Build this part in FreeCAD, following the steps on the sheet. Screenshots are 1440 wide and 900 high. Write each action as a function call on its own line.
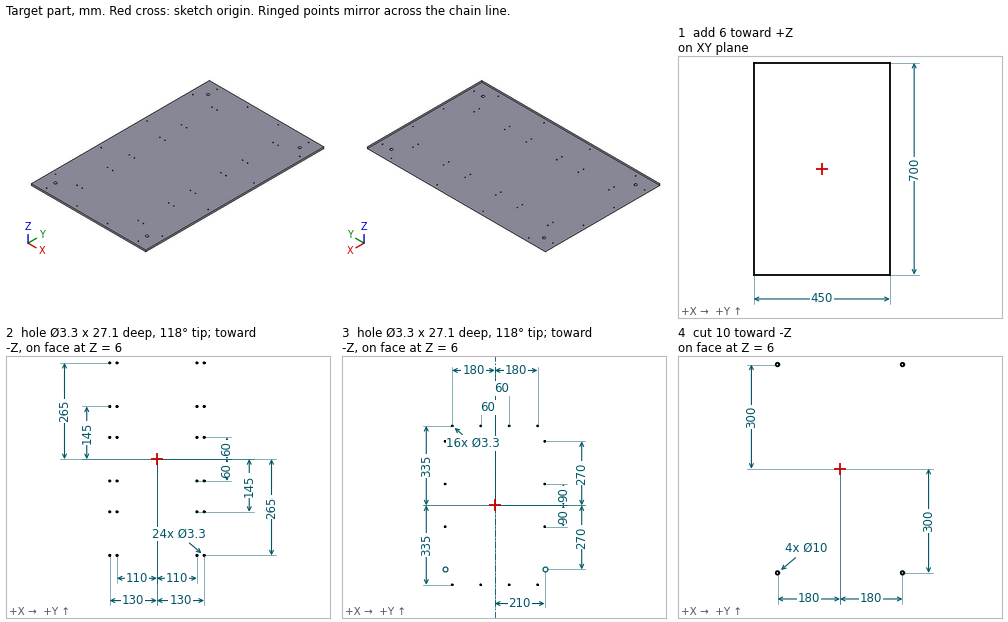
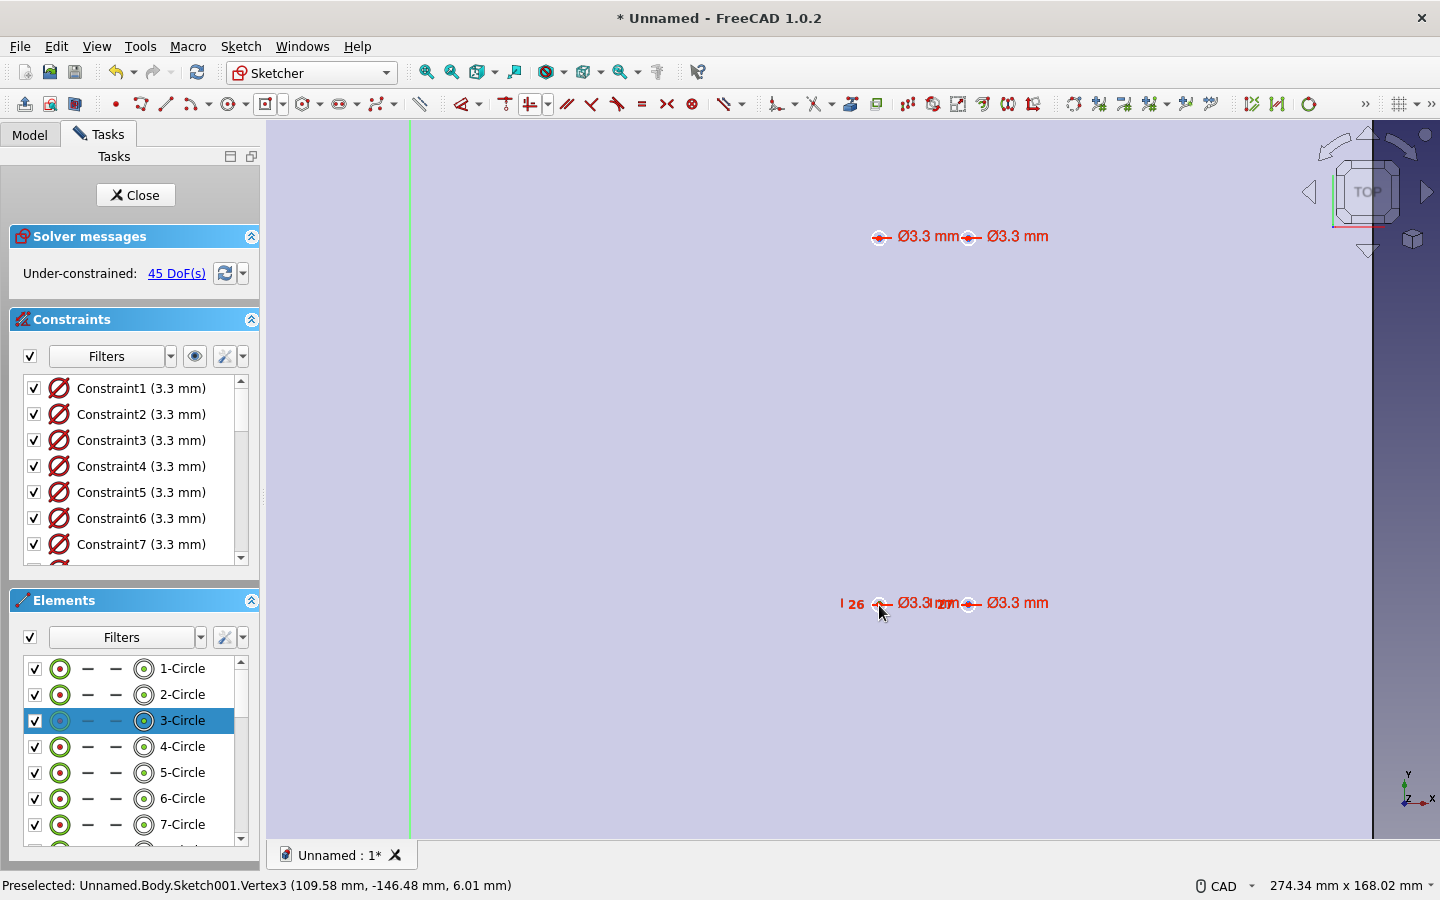
scroll(879, 606, down, 8)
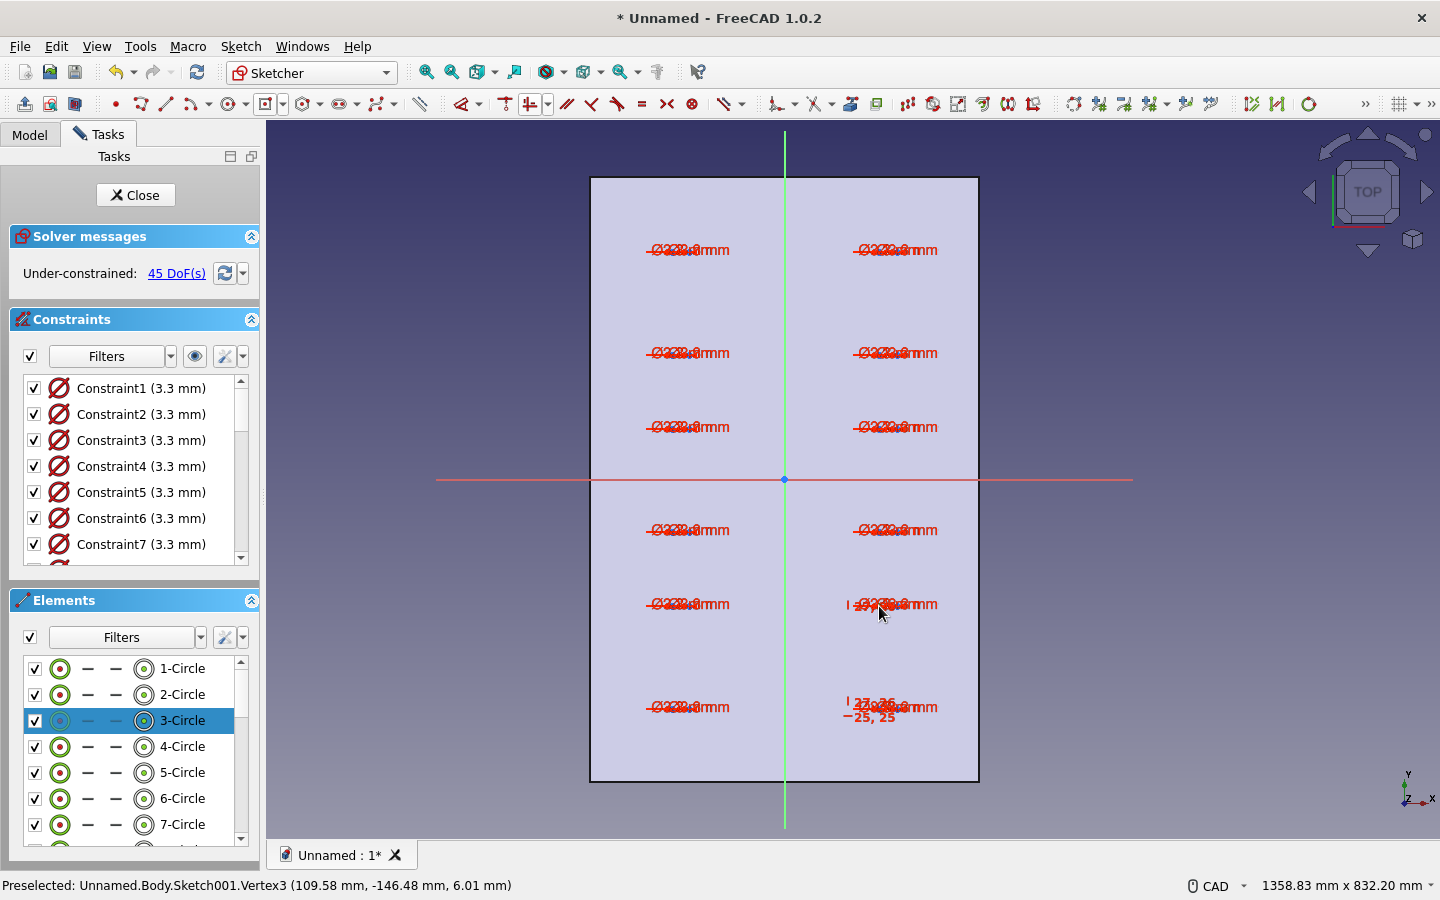
click(897, 606)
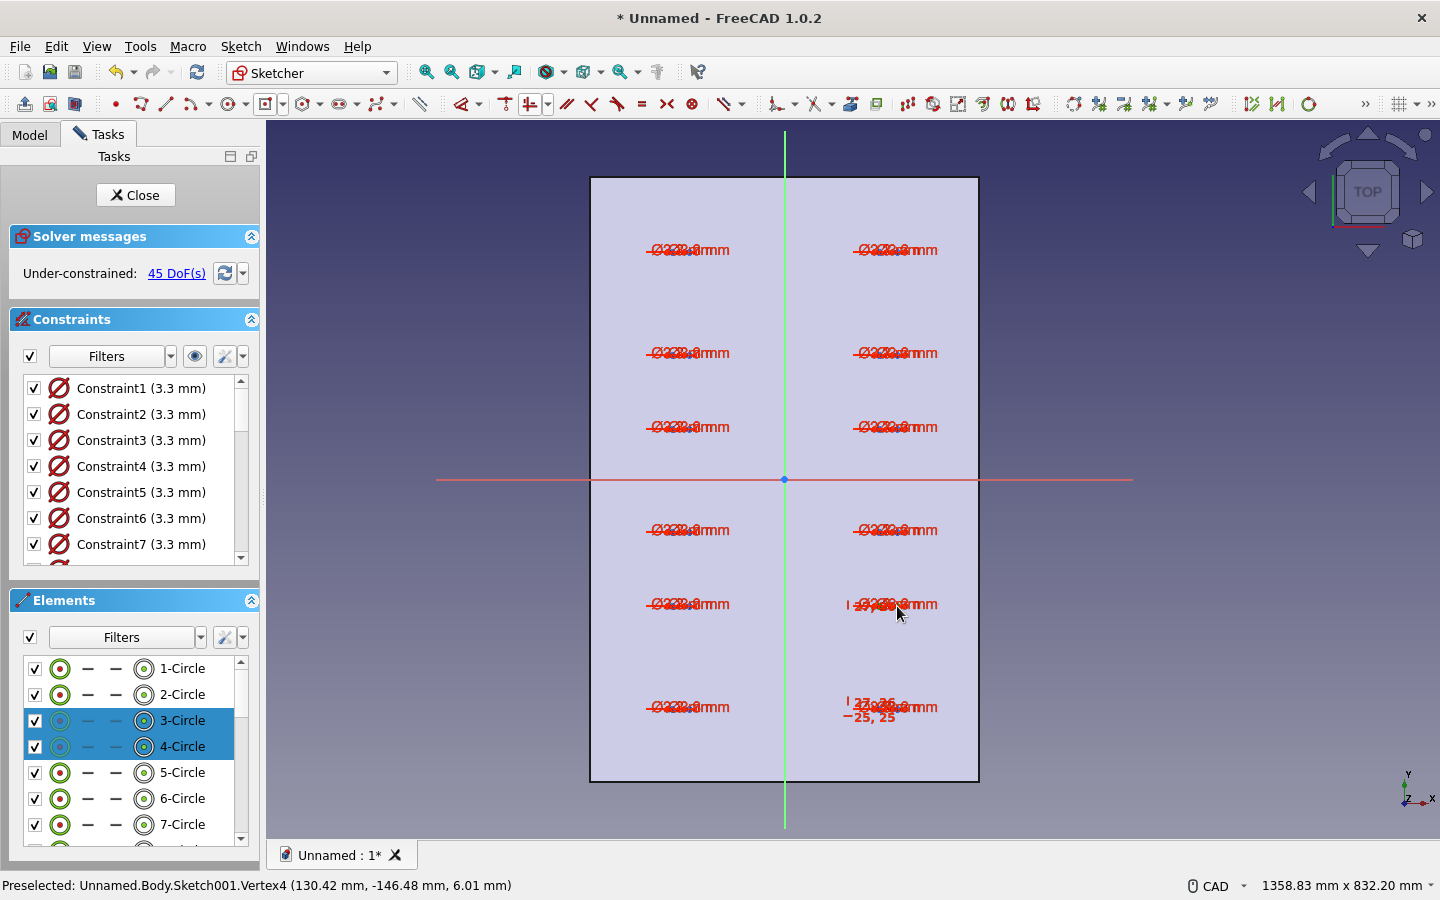
click(548, 104)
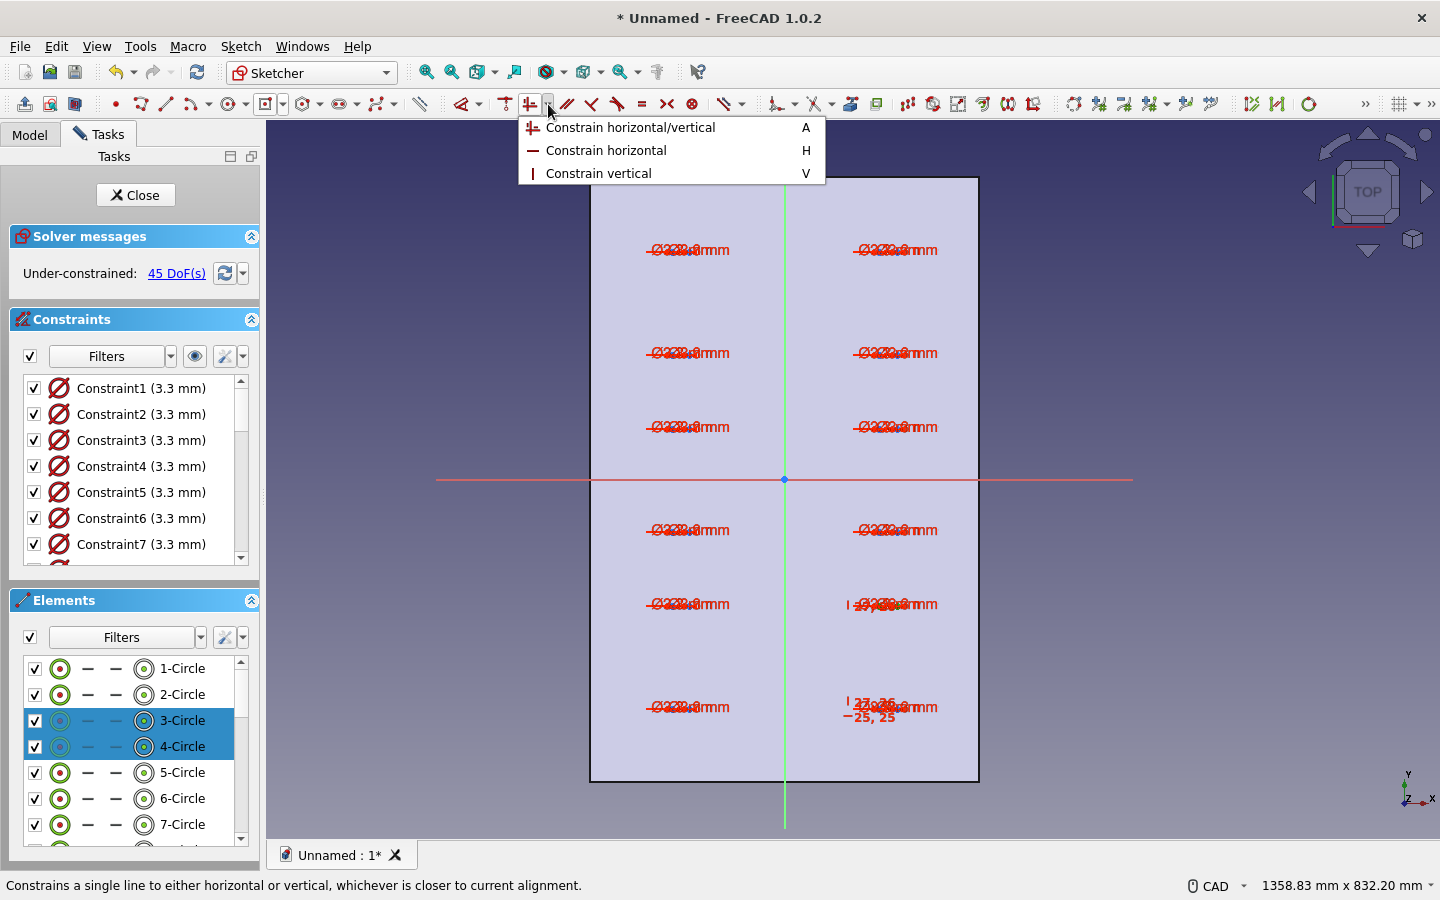
click(672, 150)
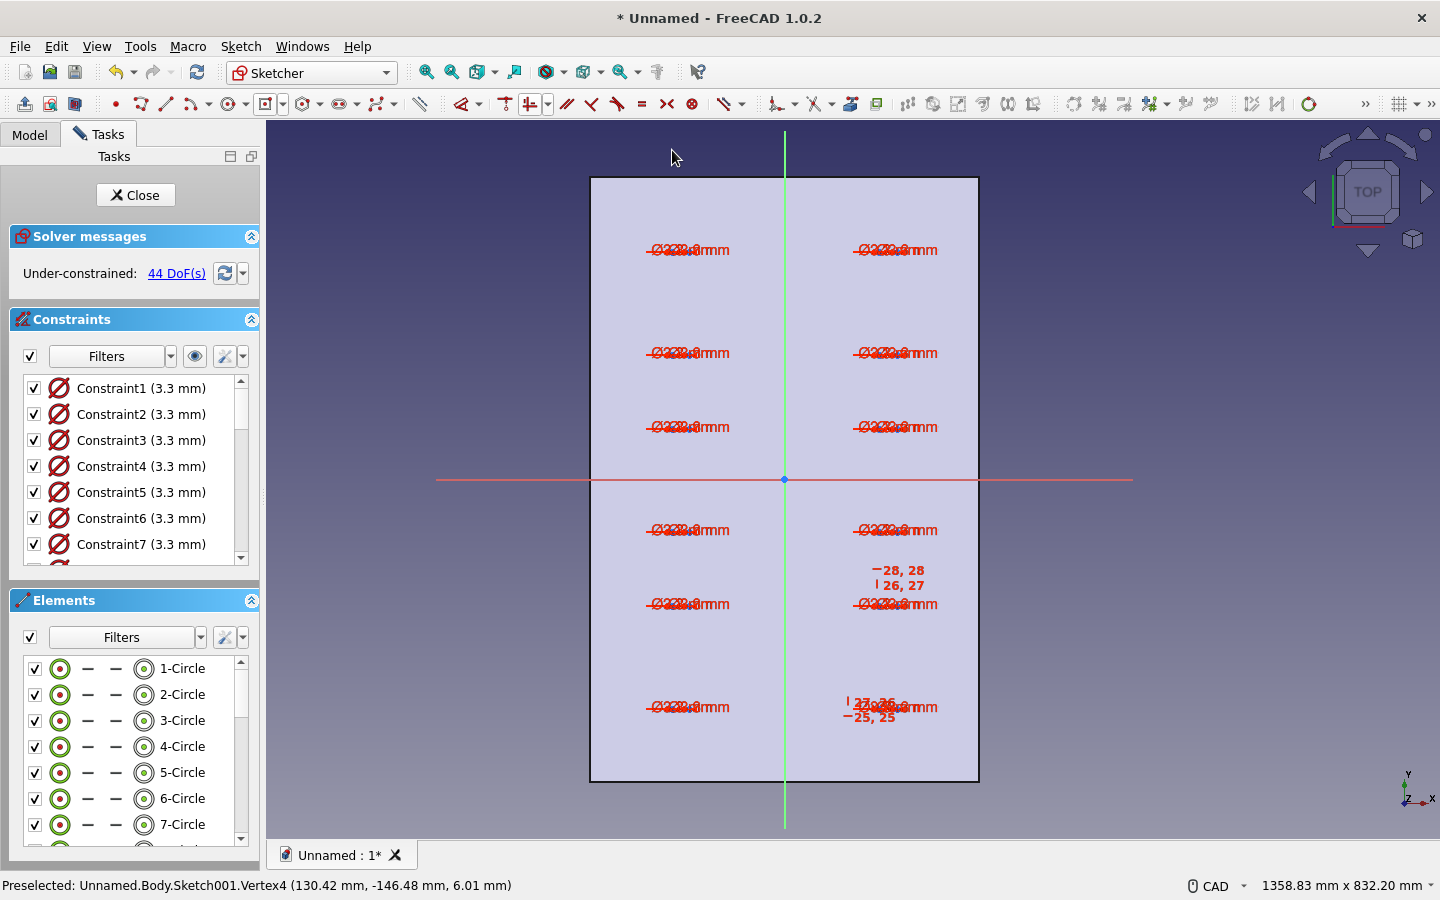
click(879, 606)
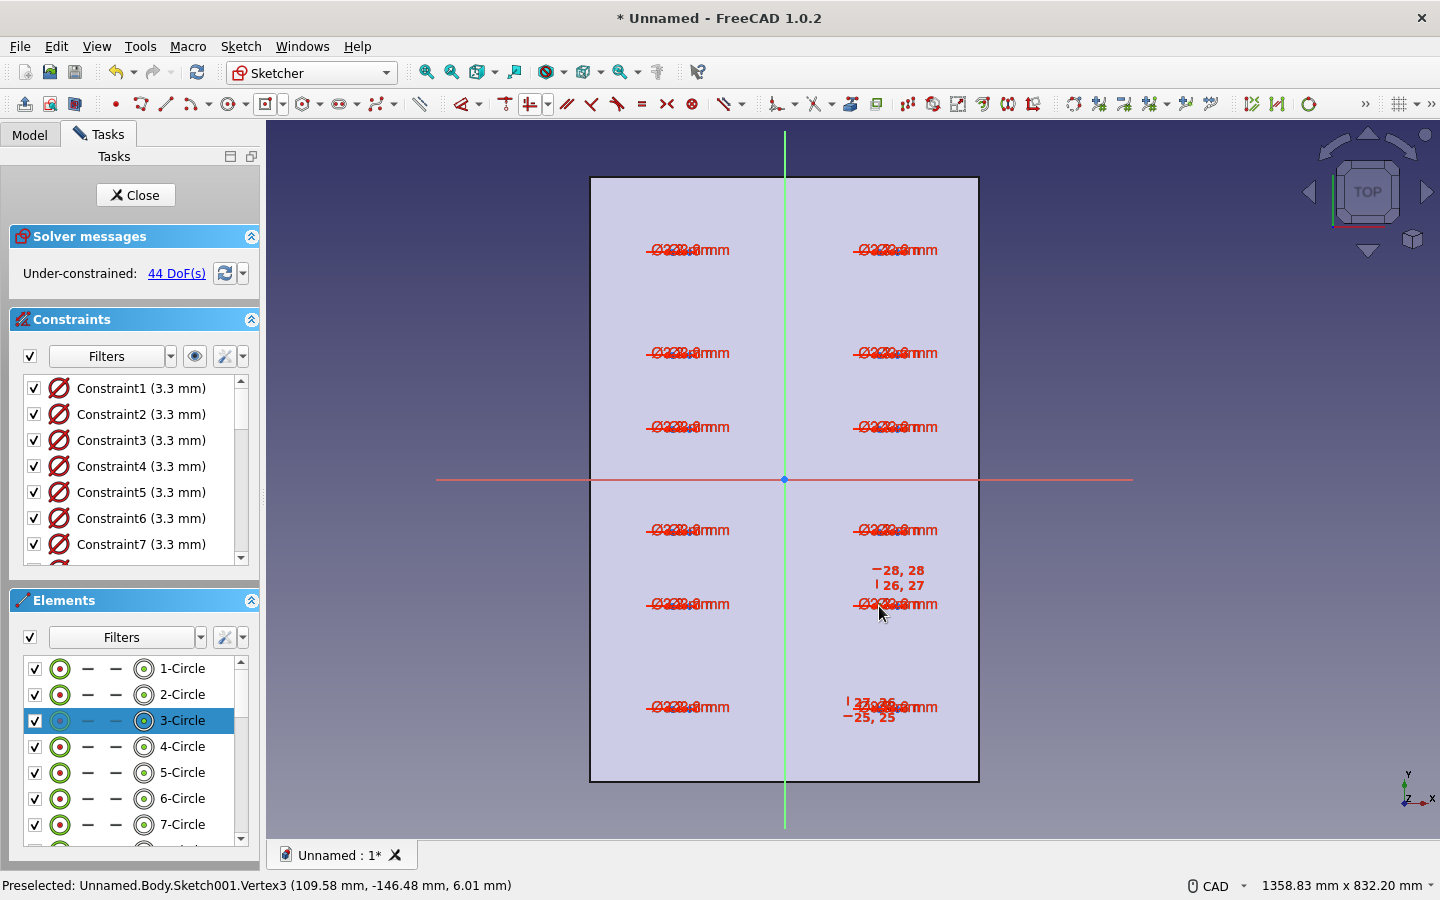
click(879, 532)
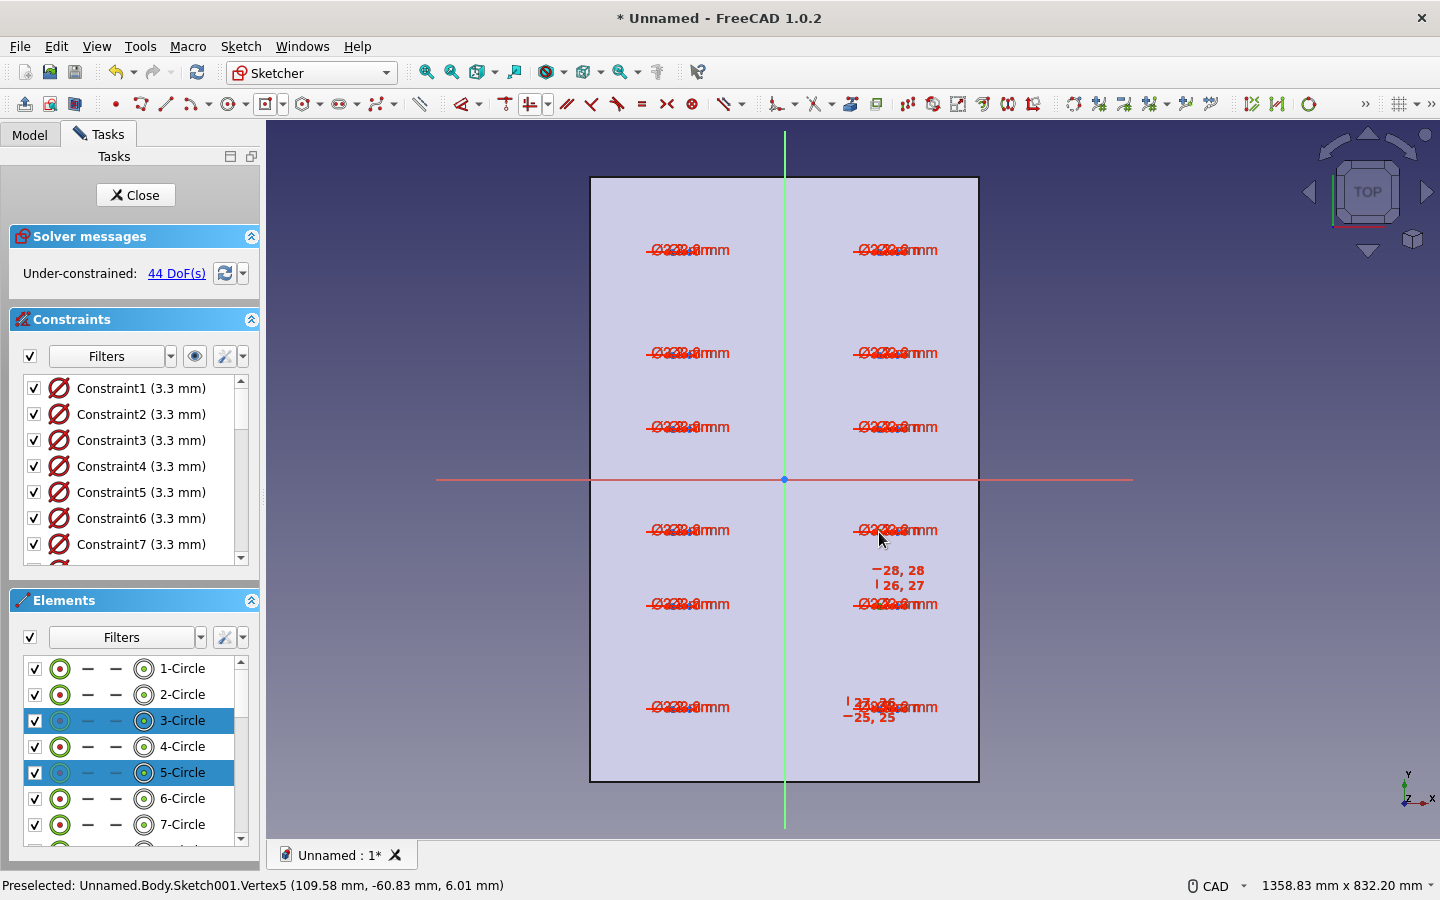
click(548, 104)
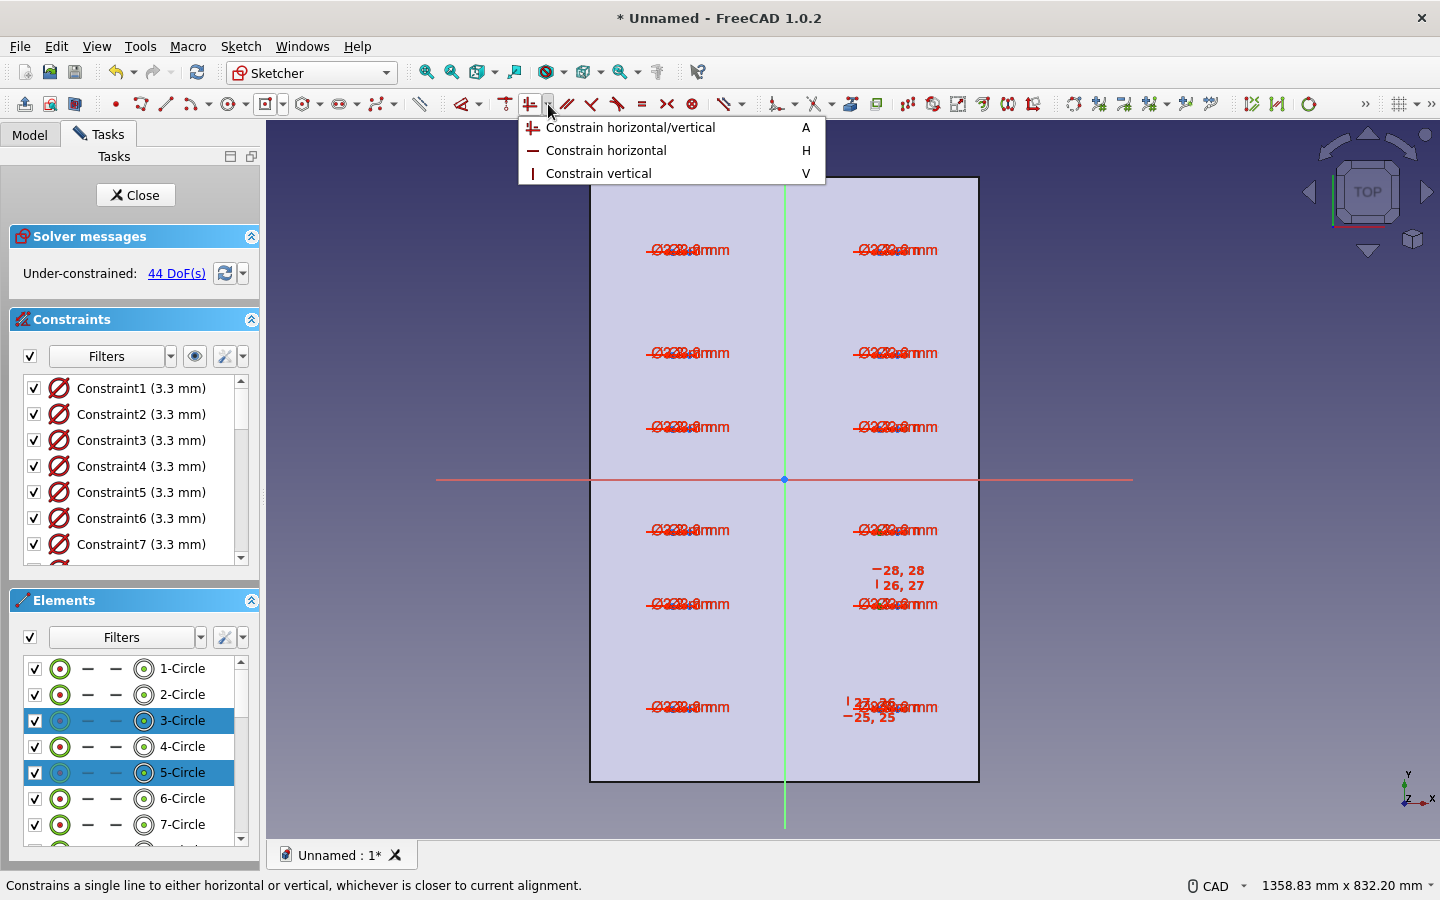
click(672, 174)